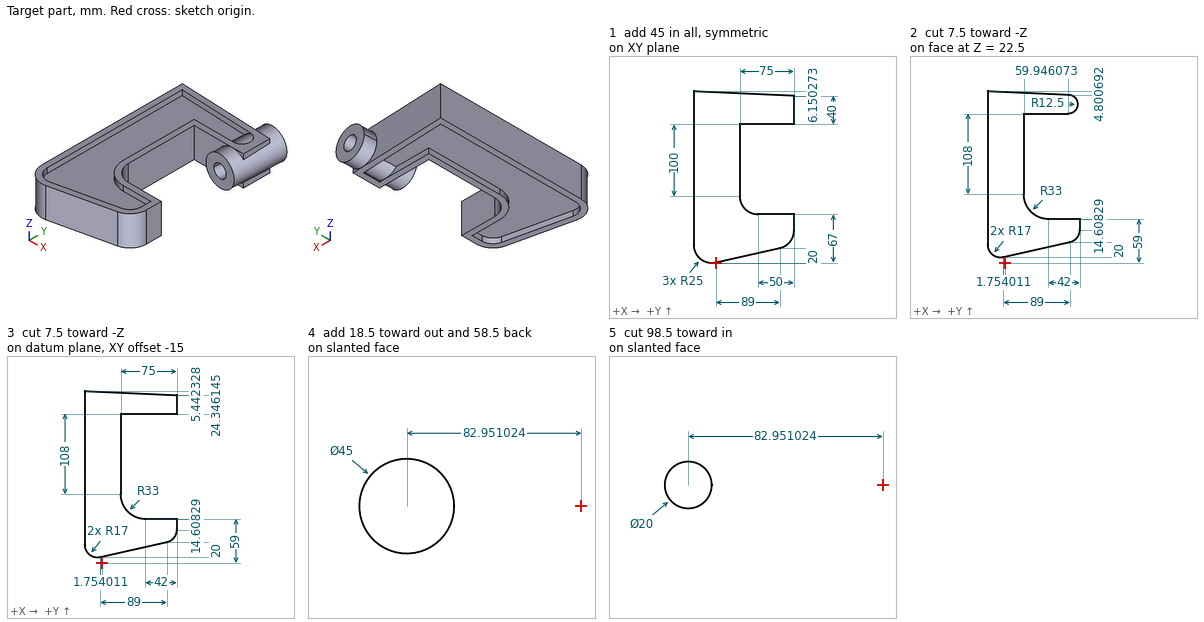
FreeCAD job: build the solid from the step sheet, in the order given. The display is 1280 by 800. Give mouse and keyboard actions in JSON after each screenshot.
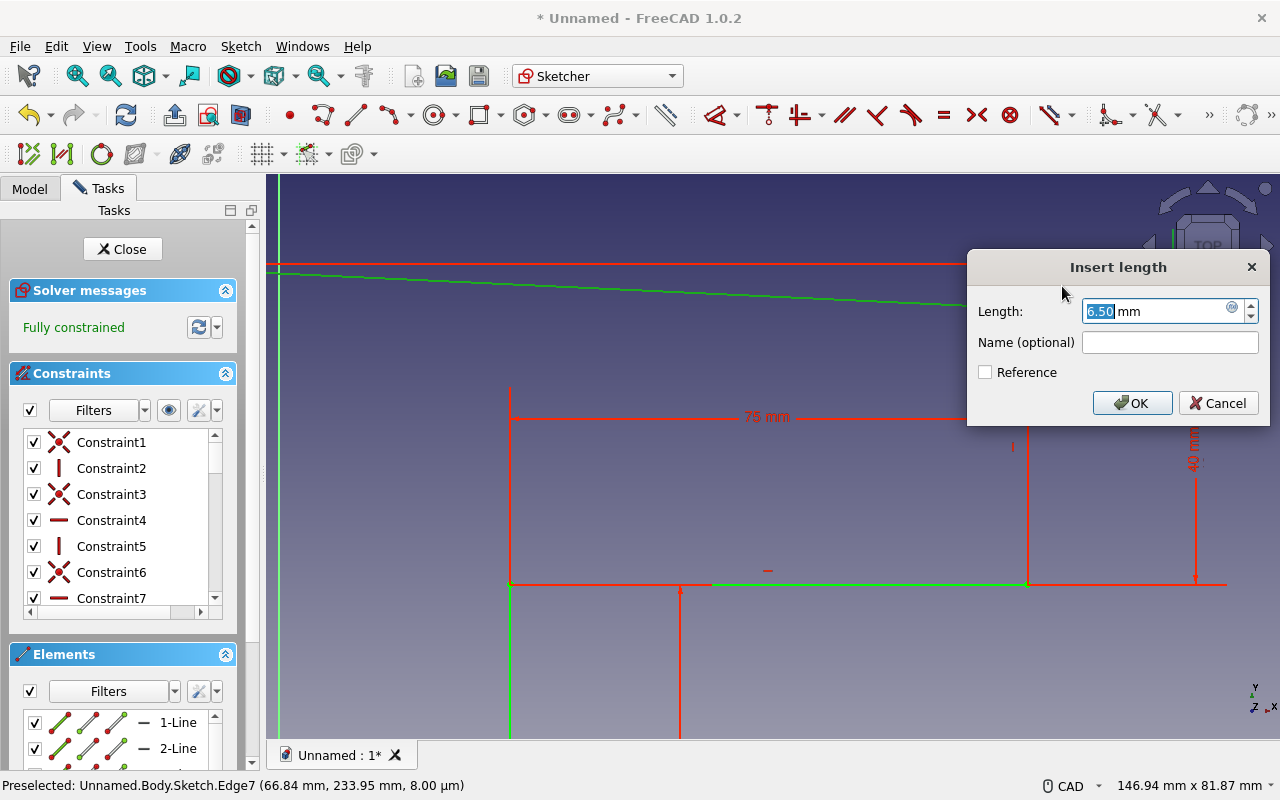
{"action": "type", "text": "6.150273"}
{"action": "key", "text": "Return"}
{"action": "key", "text": "Escape"}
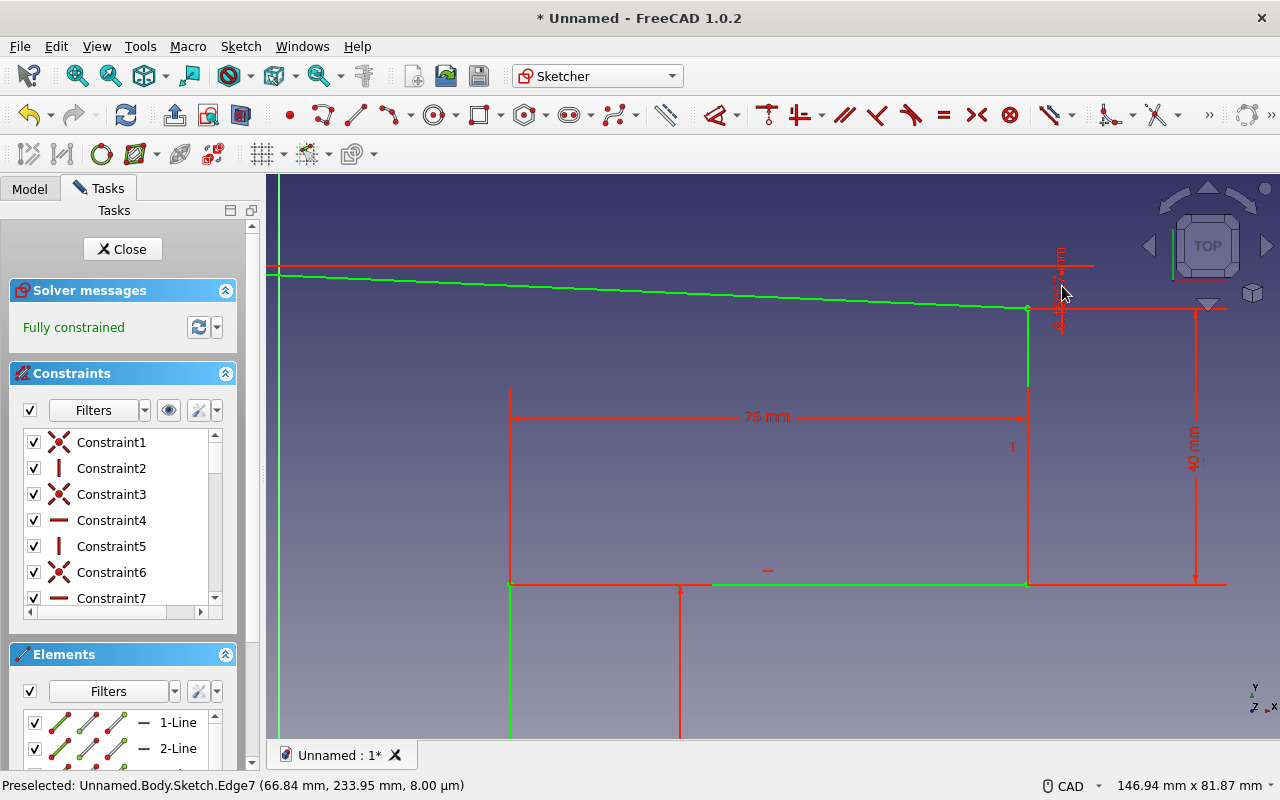
{"action": "left_click", "coordinate": [123, 249]}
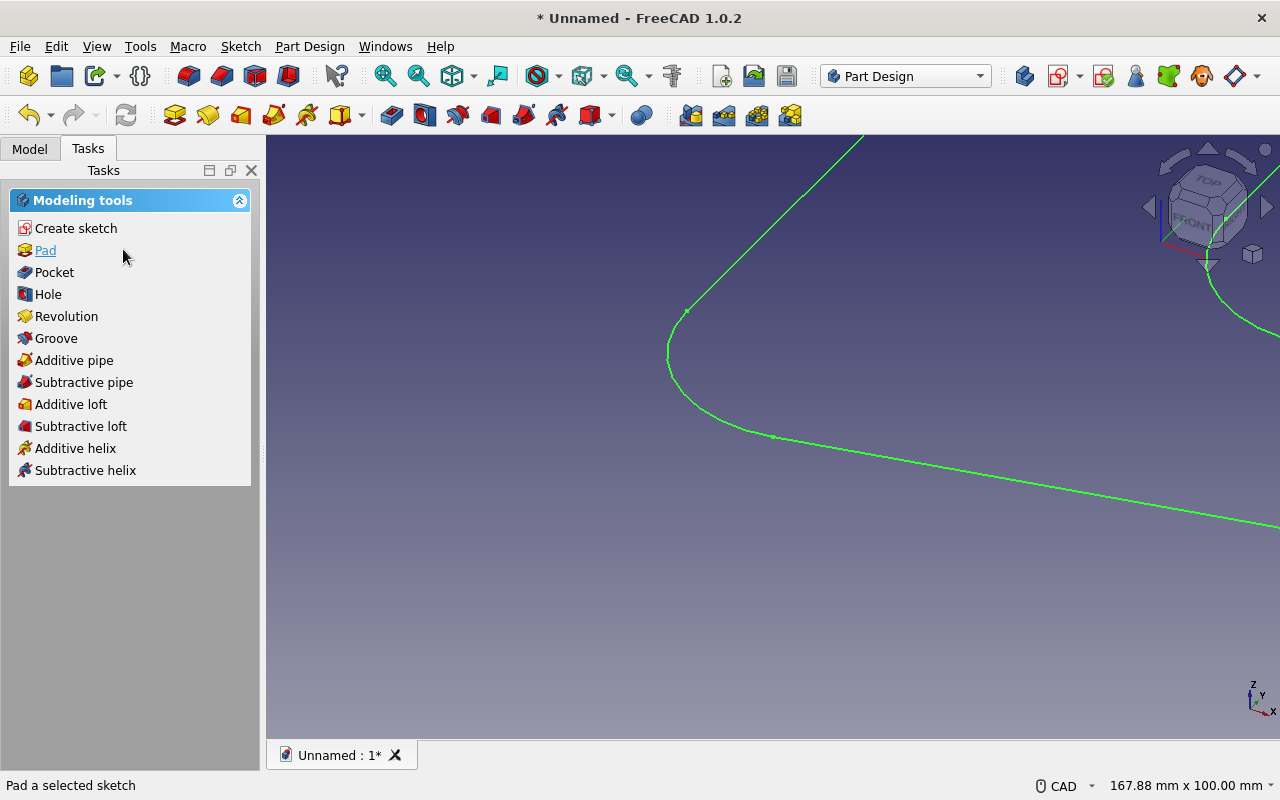
{"action": "left_click", "coordinate": [175, 116]}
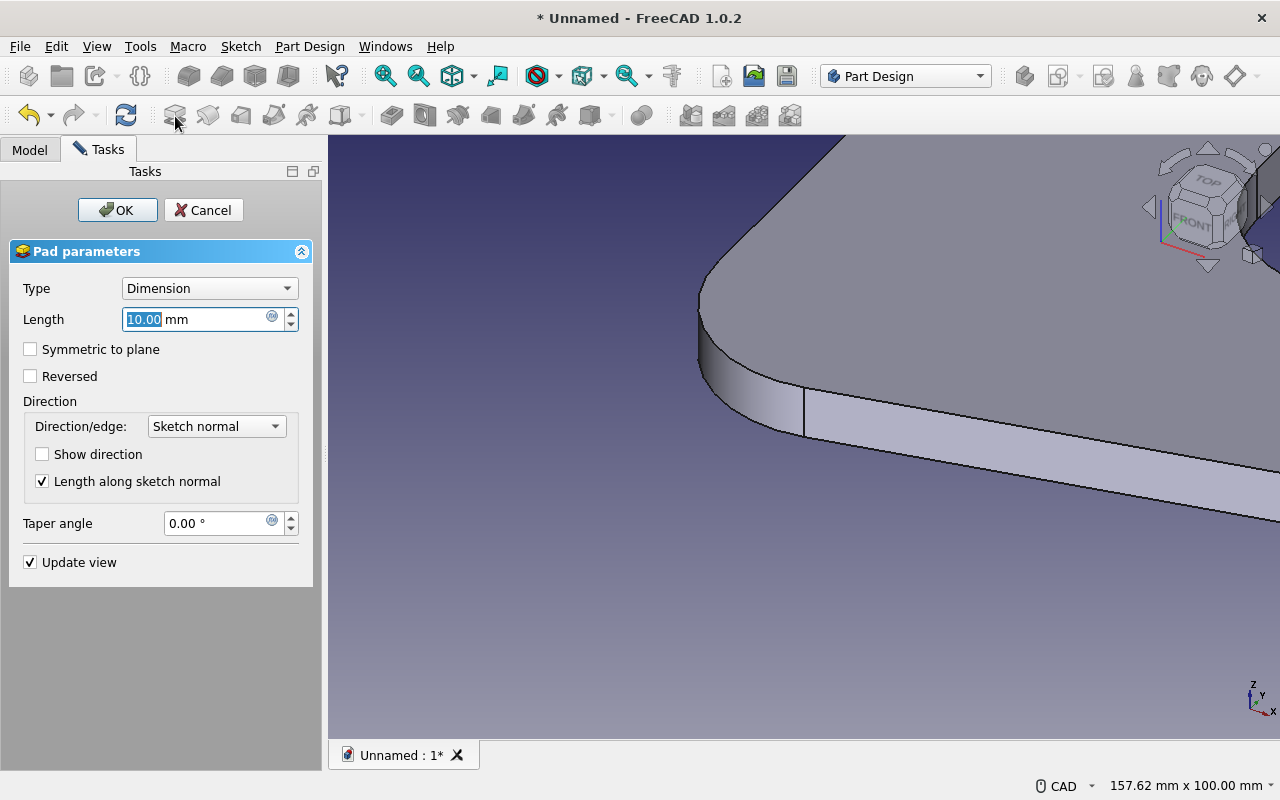
{"action": "type", "text": "45"}
{"action": "key", "text": "Tab"}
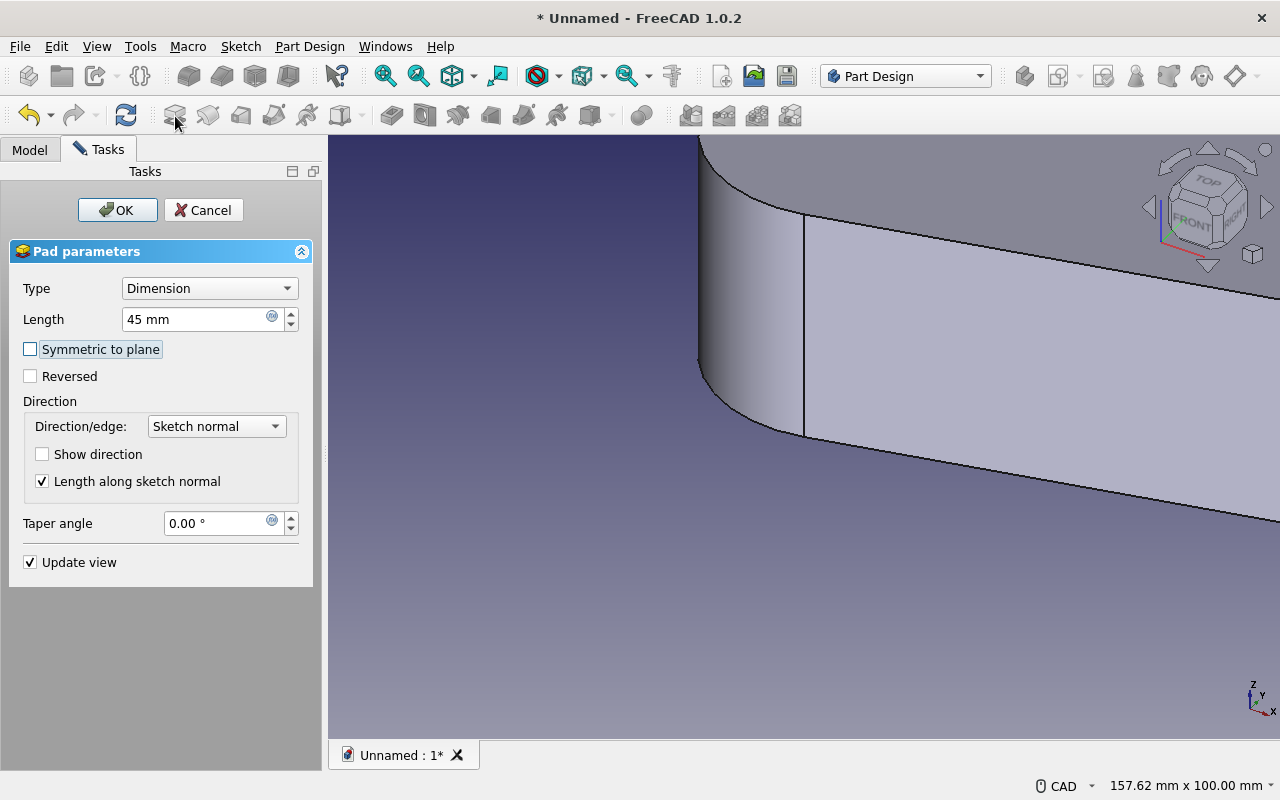
{"action": "left_click", "coordinate": [31, 349]}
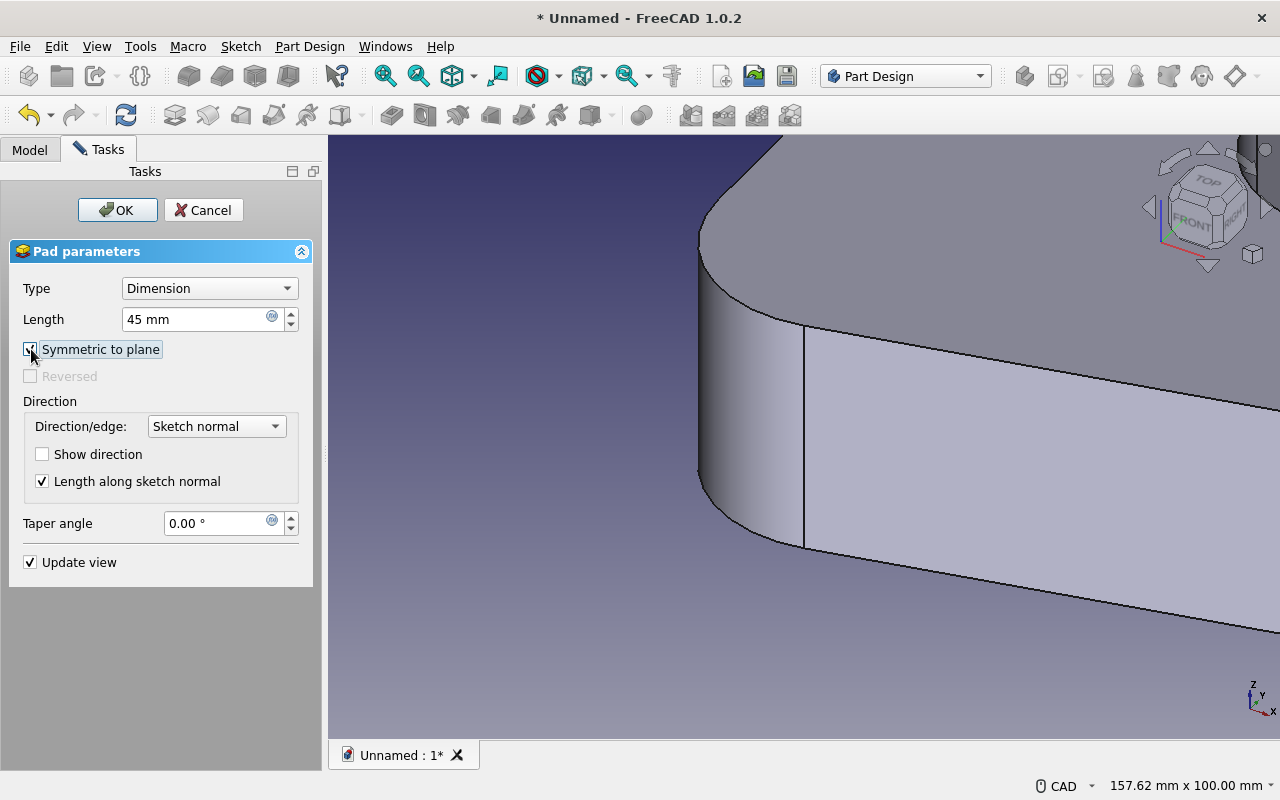
{"action": "left_click", "coordinate": [118, 210]}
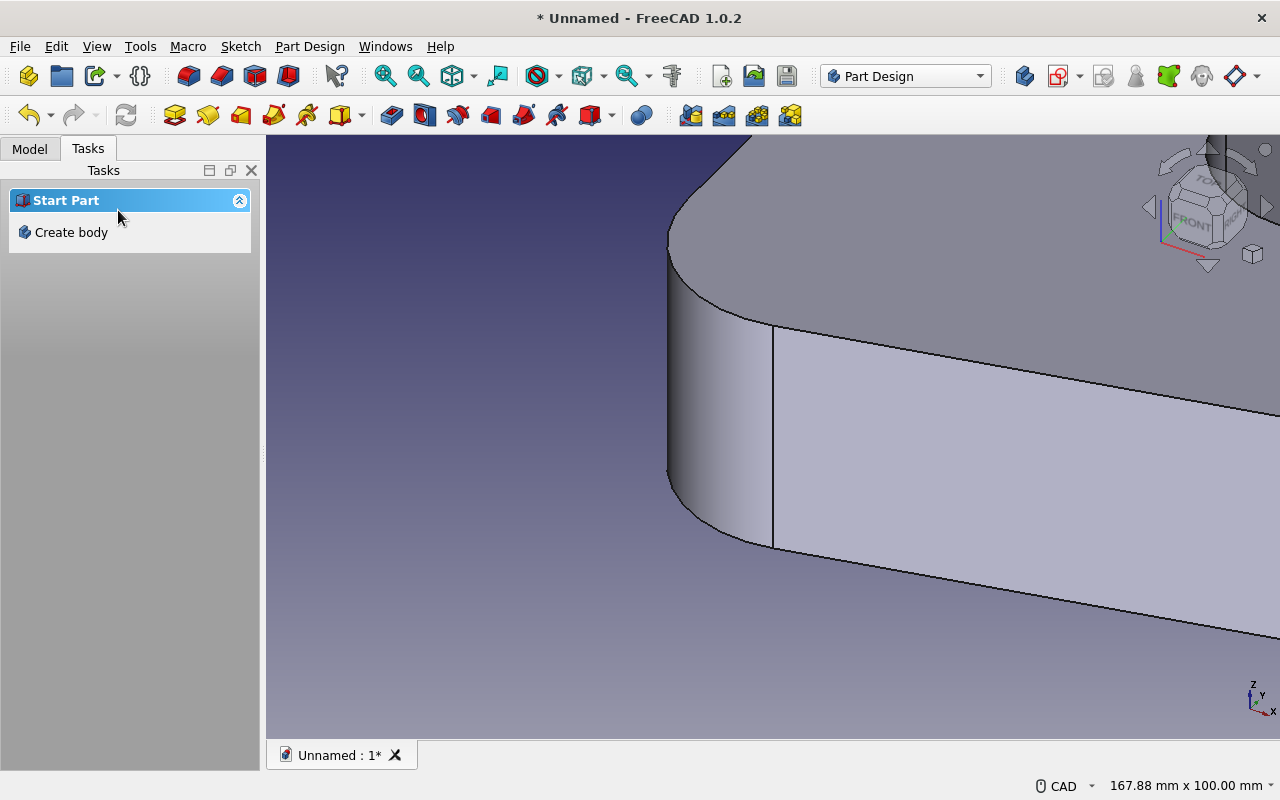
{"action": "left_click", "coordinate": [386, 76]}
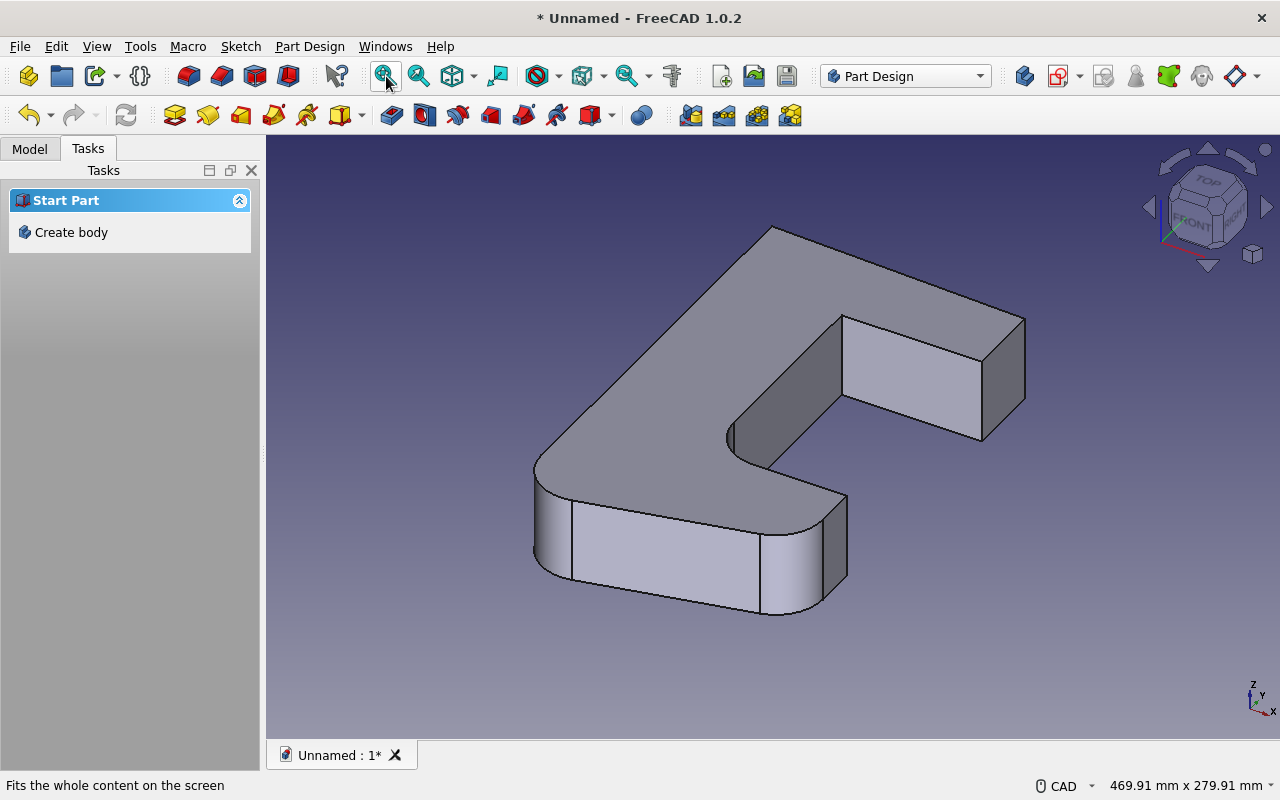
{"action": "left_click", "coordinate": [662, 457]}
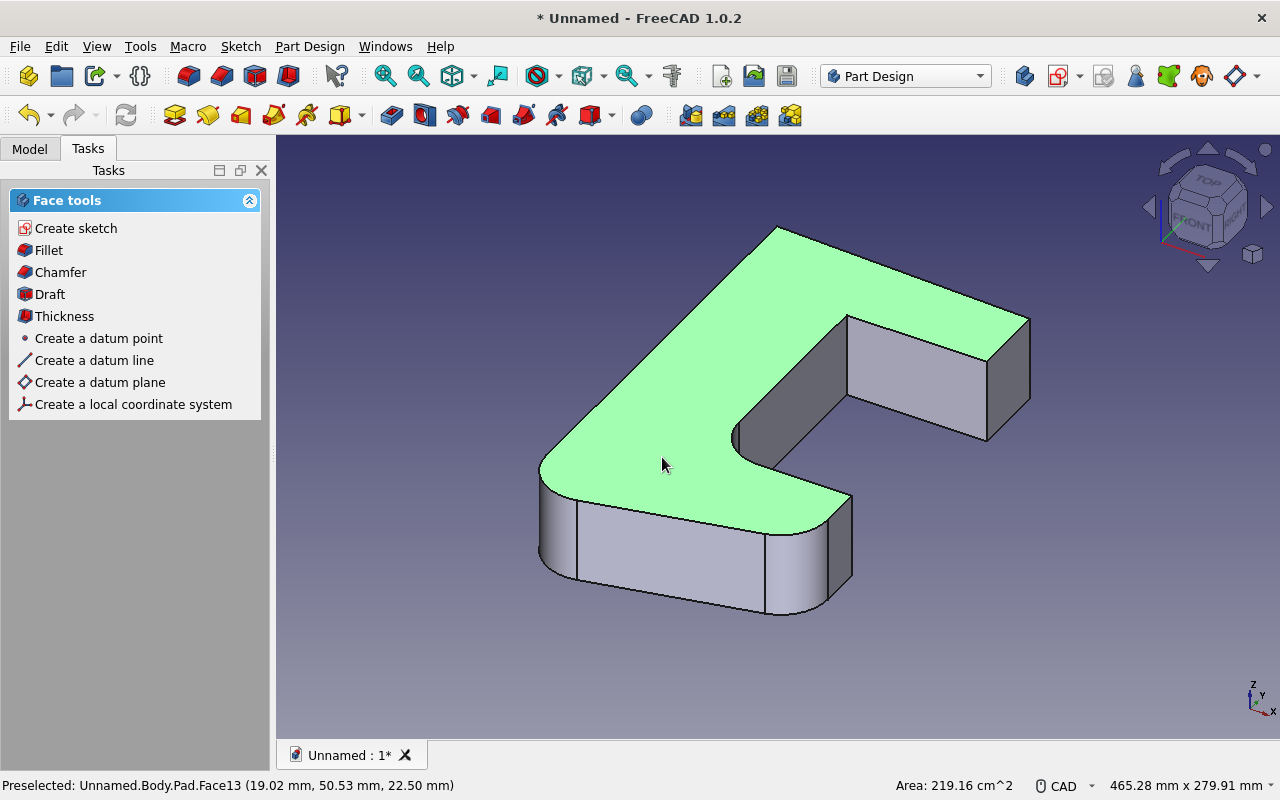
{"action": "left_click", "coordinate": [1058, 76]}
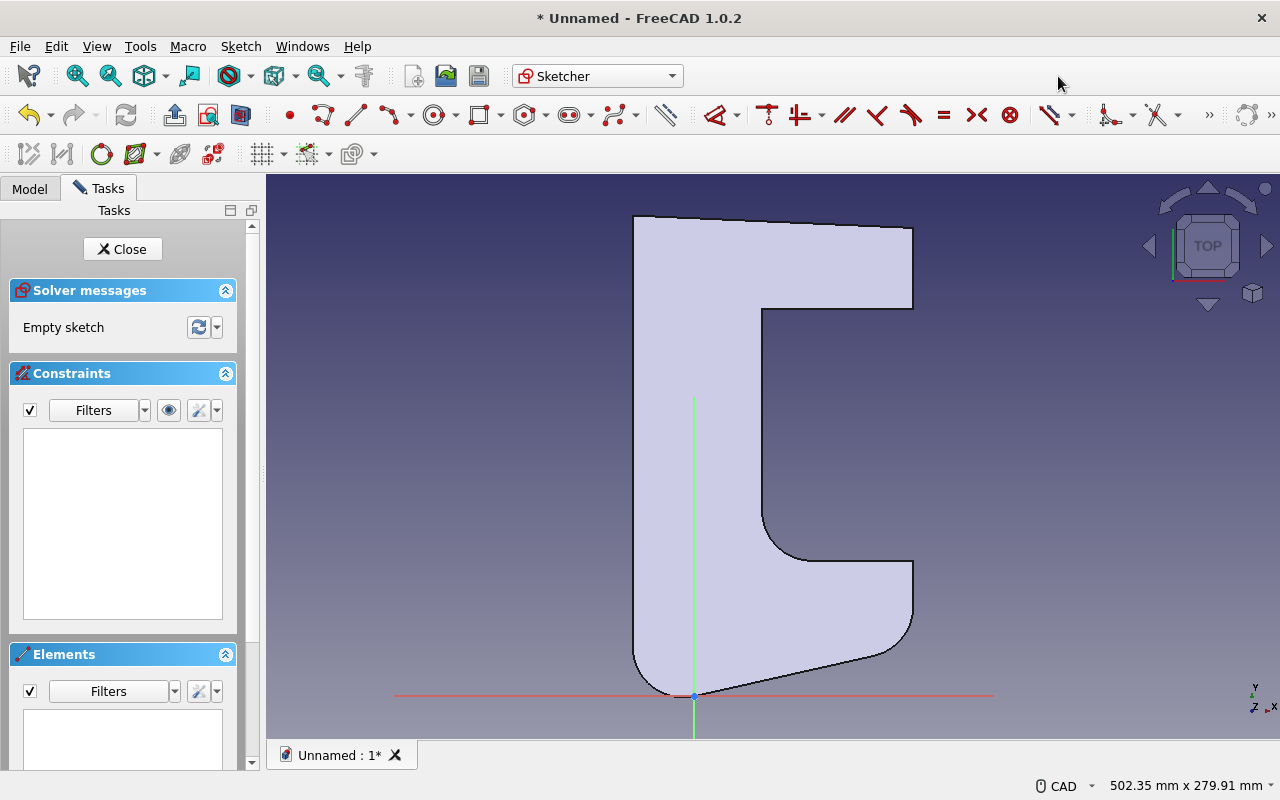
{"action": "scroll", "coordinate": [395, 421], "scroll_direction": "down", "scroll_amount": 1}